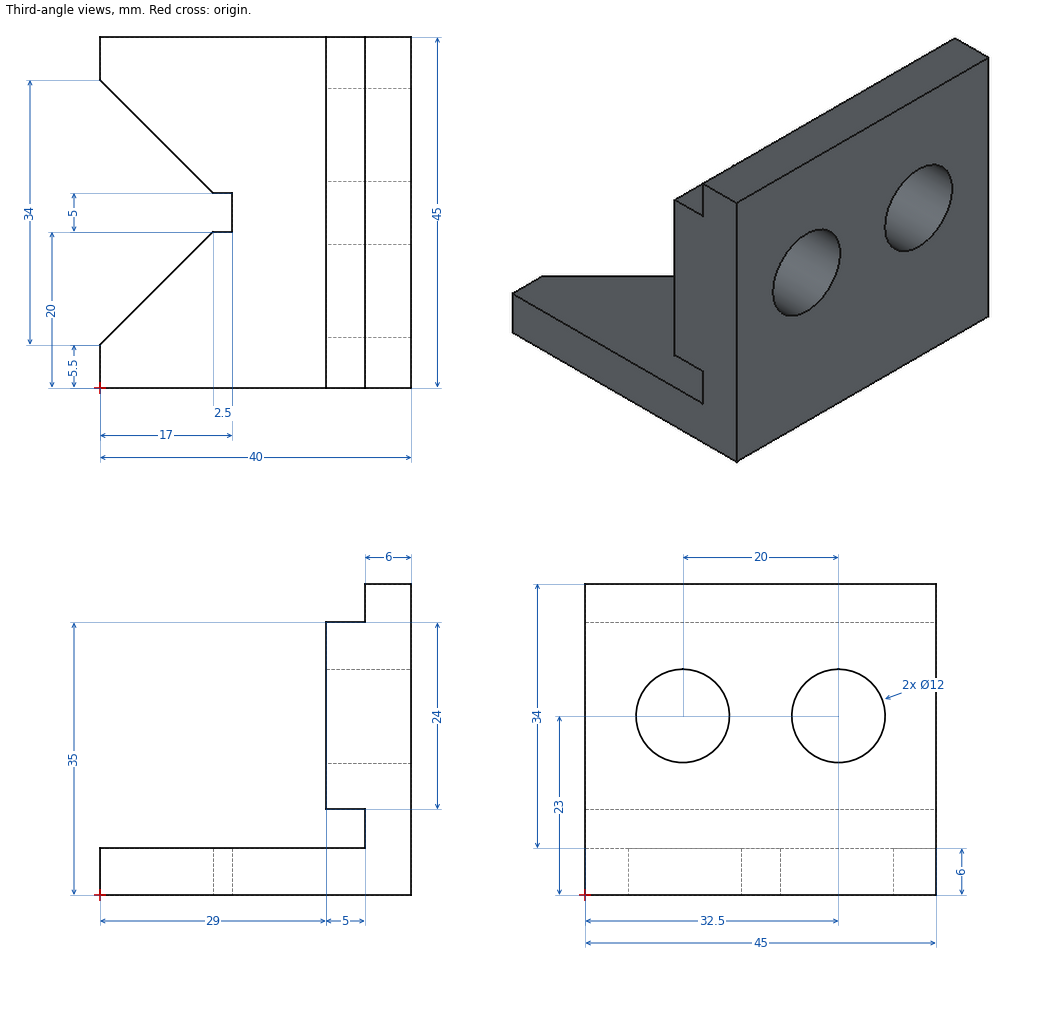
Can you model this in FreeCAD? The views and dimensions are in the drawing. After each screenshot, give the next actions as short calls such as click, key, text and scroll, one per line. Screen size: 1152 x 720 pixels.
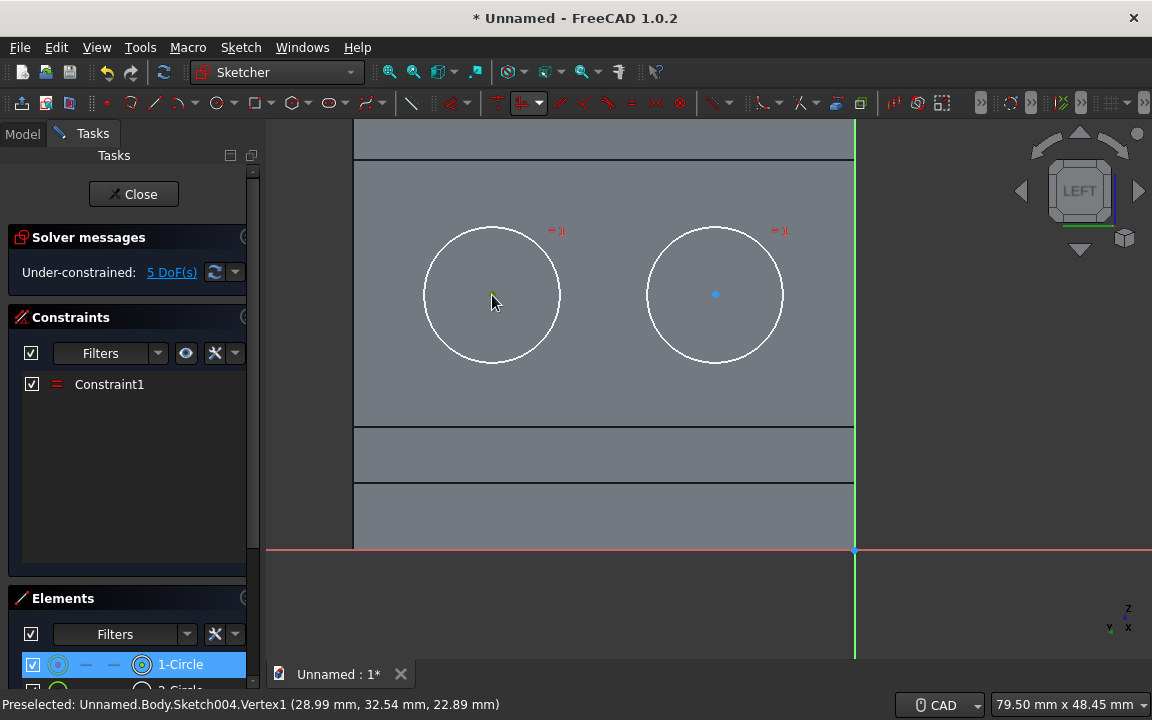
click(715, 295)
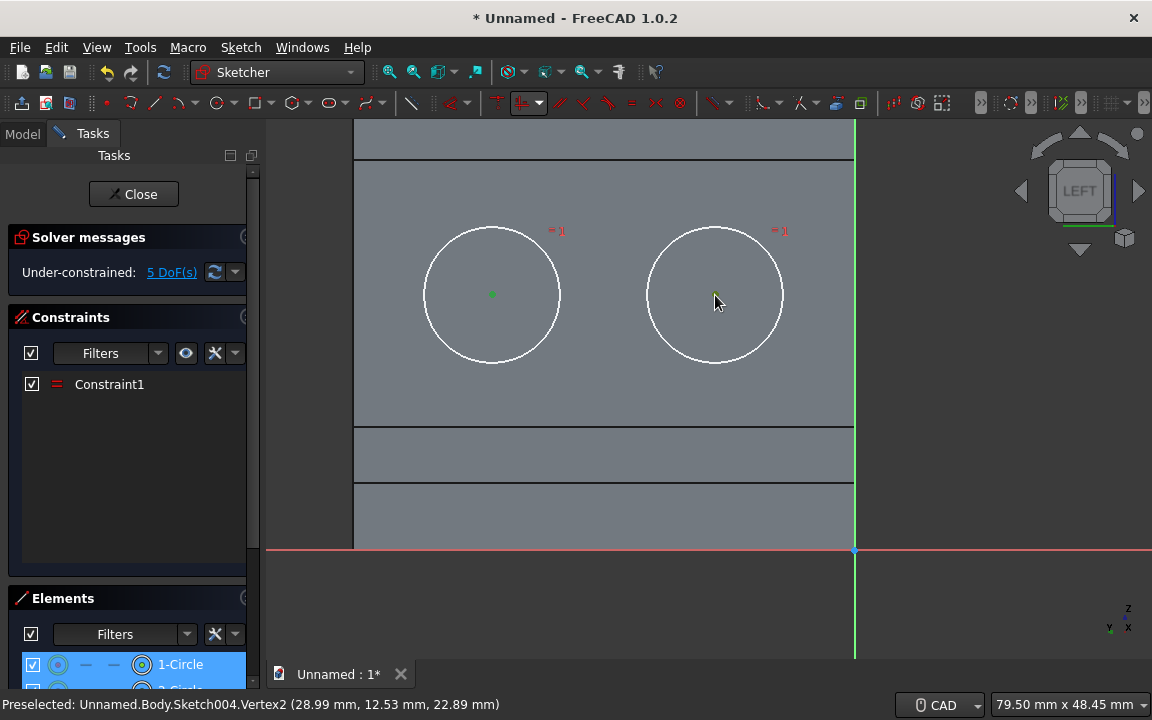
click(542, 104)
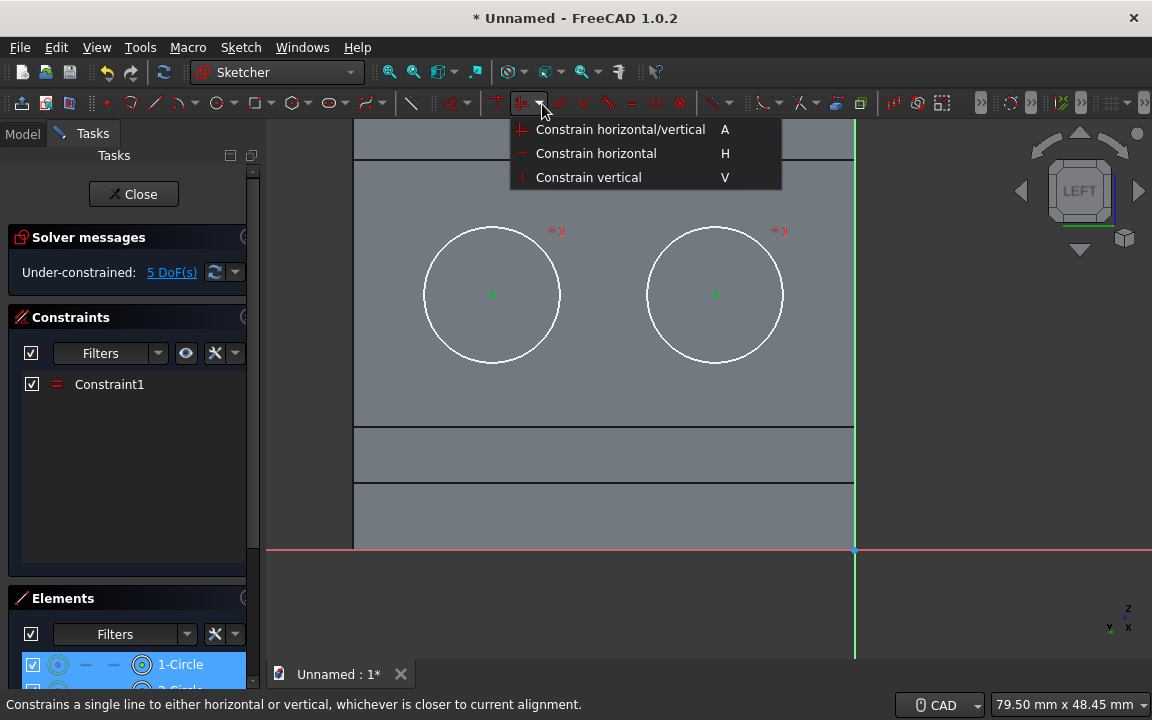
click(646, 153)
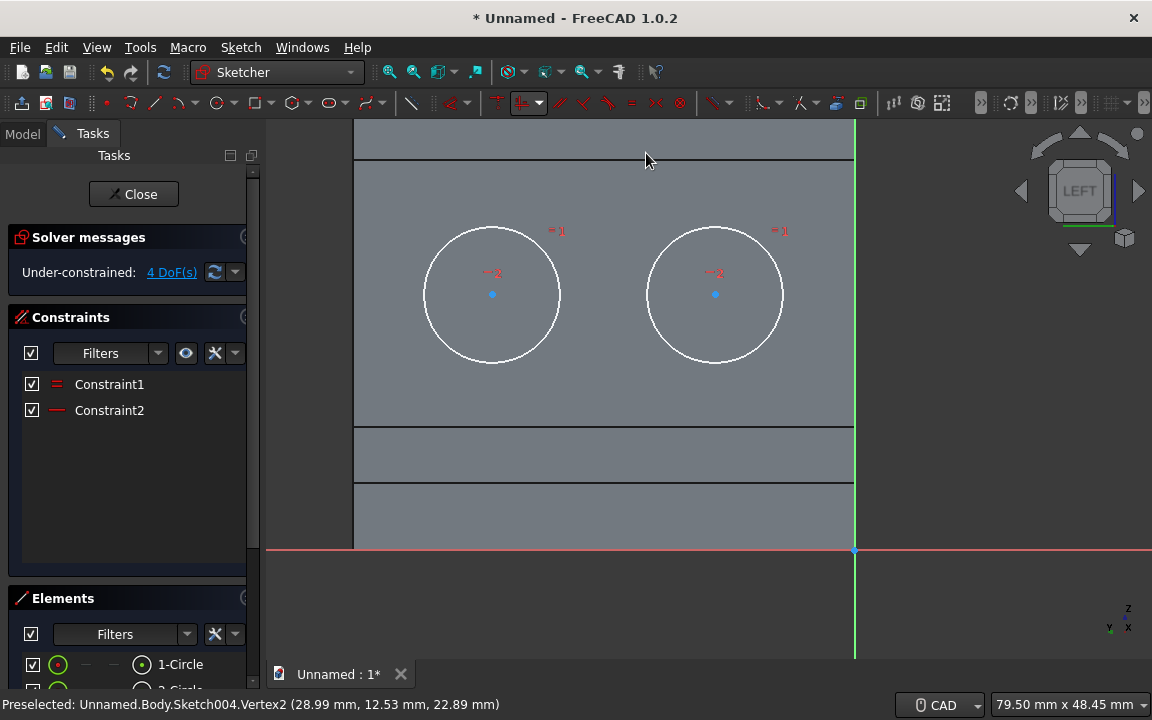
click(450, 104)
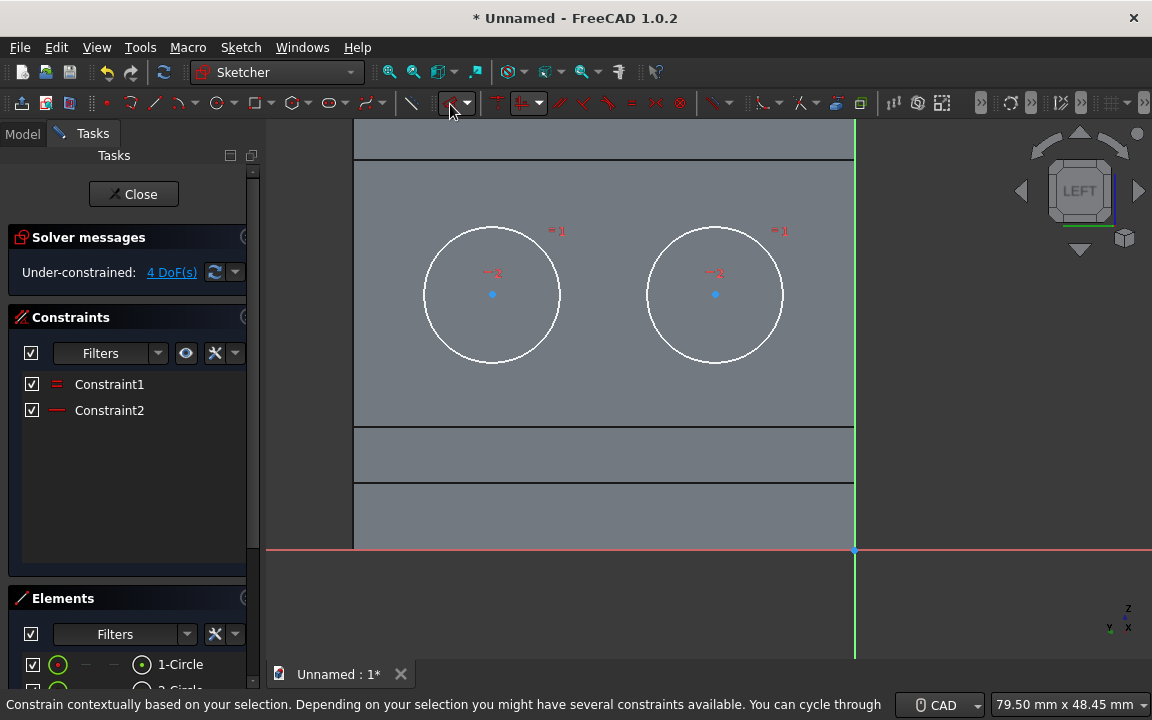
click(540, 247)
click(563, 224)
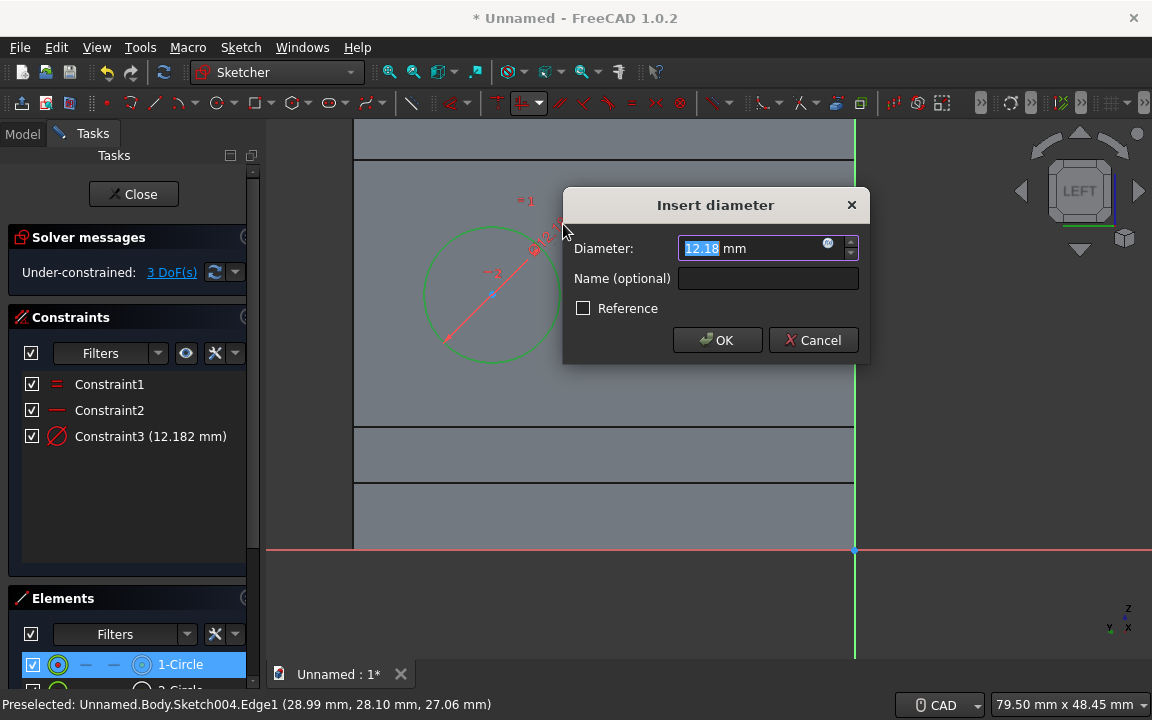
text(12)
key(Return)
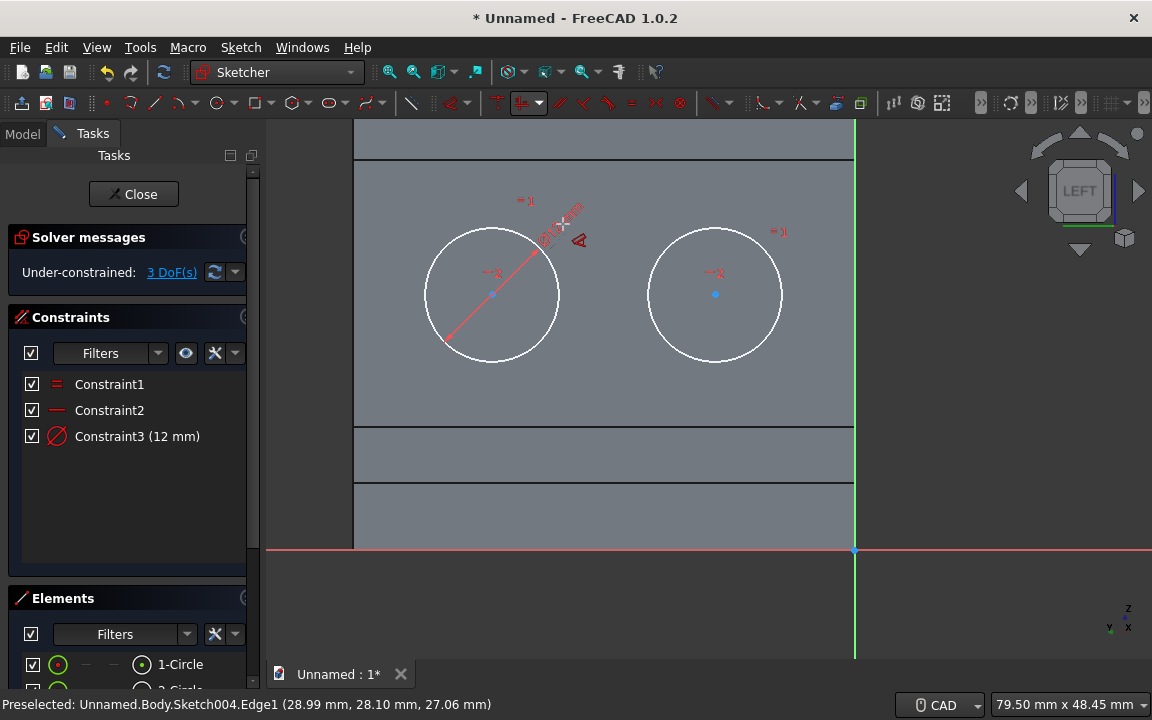
click(492, 295)
click(889, 423)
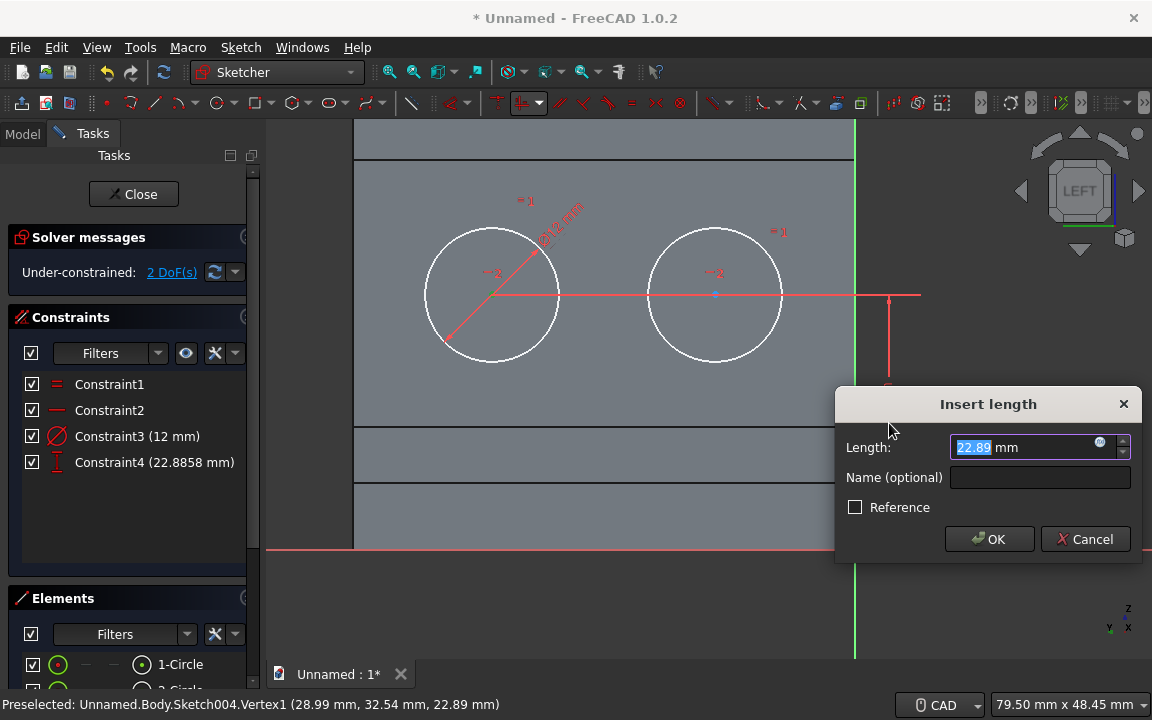
text(23)
key(Return)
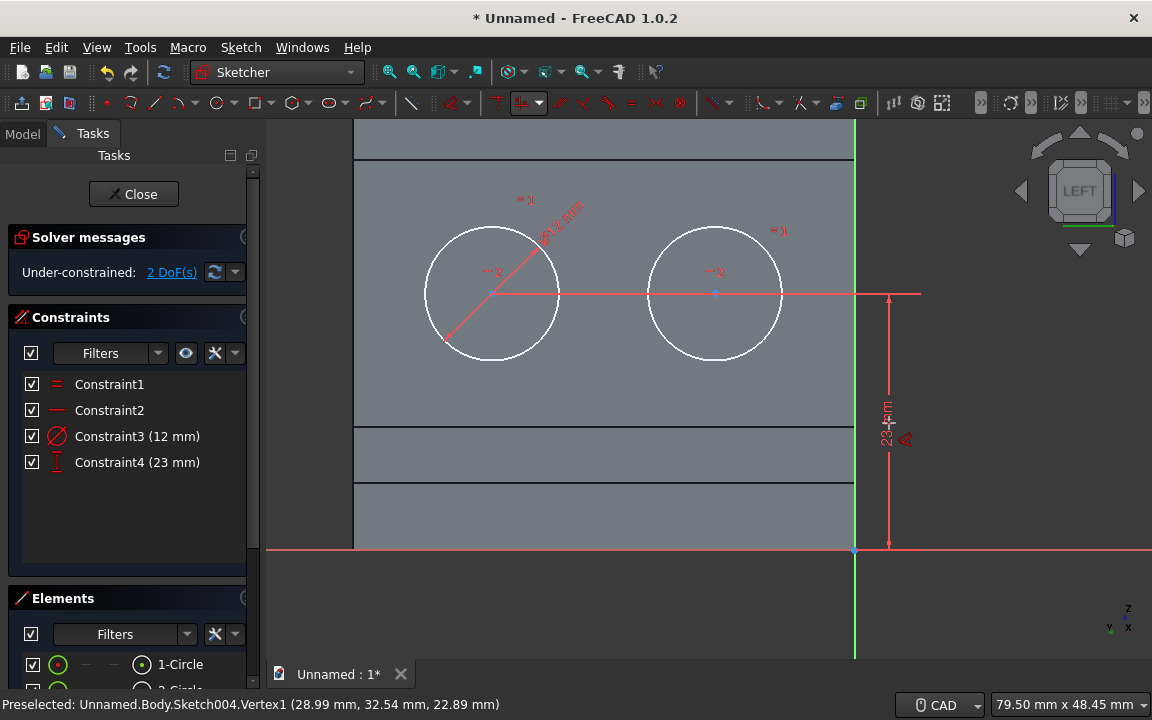
click(492, 294)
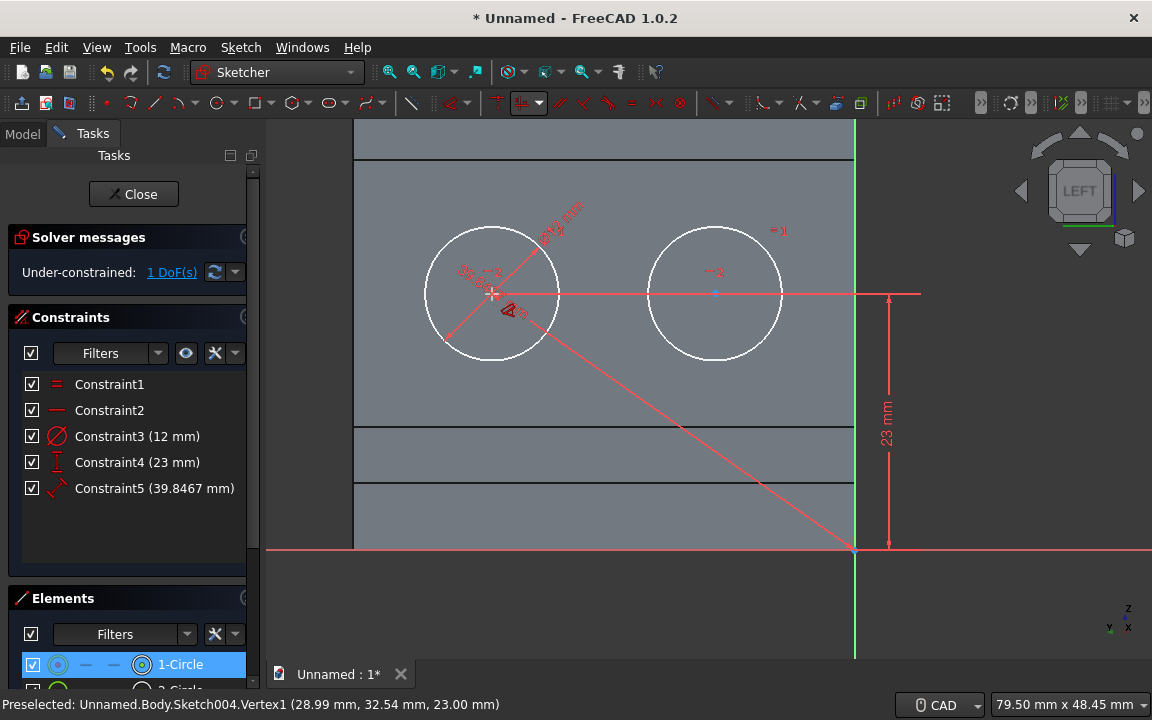
click(715, 294)
click(603, 260)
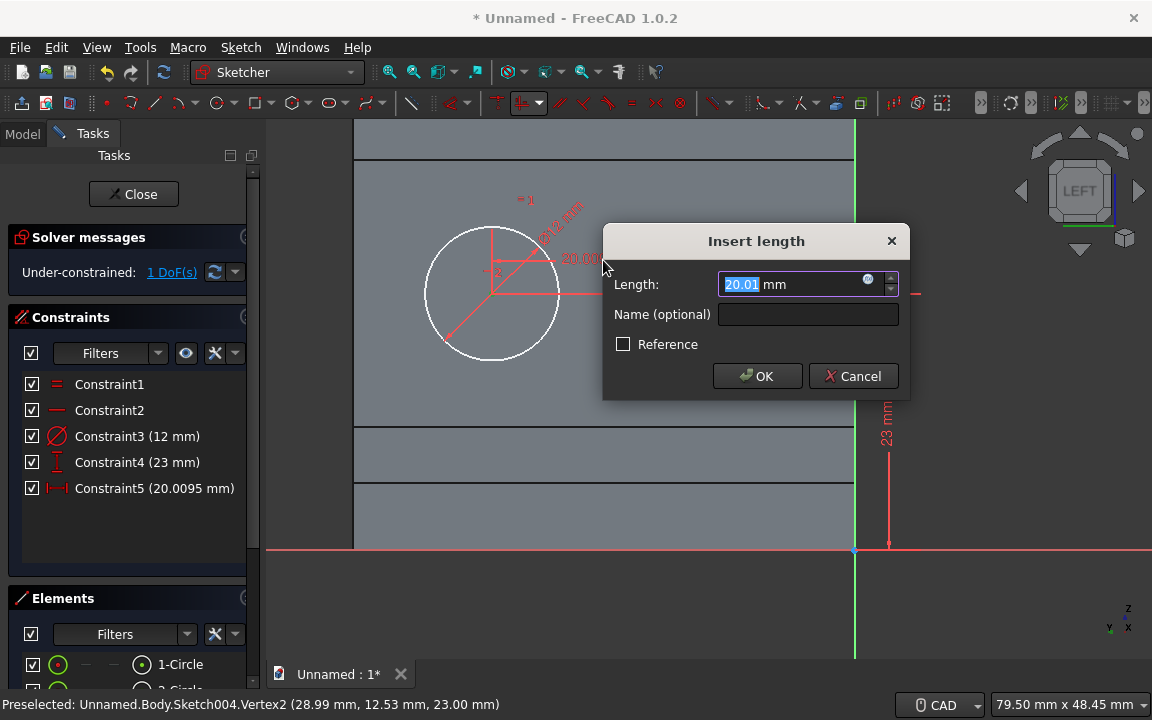
text(20)
key(Return)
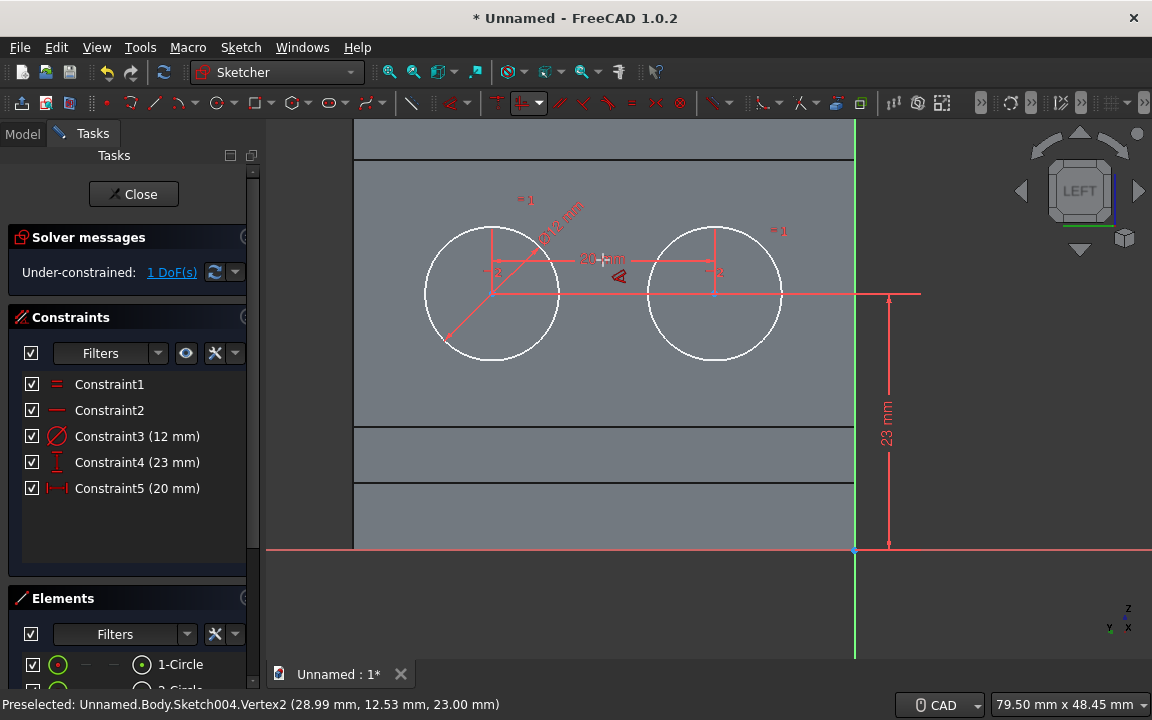
click(492, 294)
click(673, 584)